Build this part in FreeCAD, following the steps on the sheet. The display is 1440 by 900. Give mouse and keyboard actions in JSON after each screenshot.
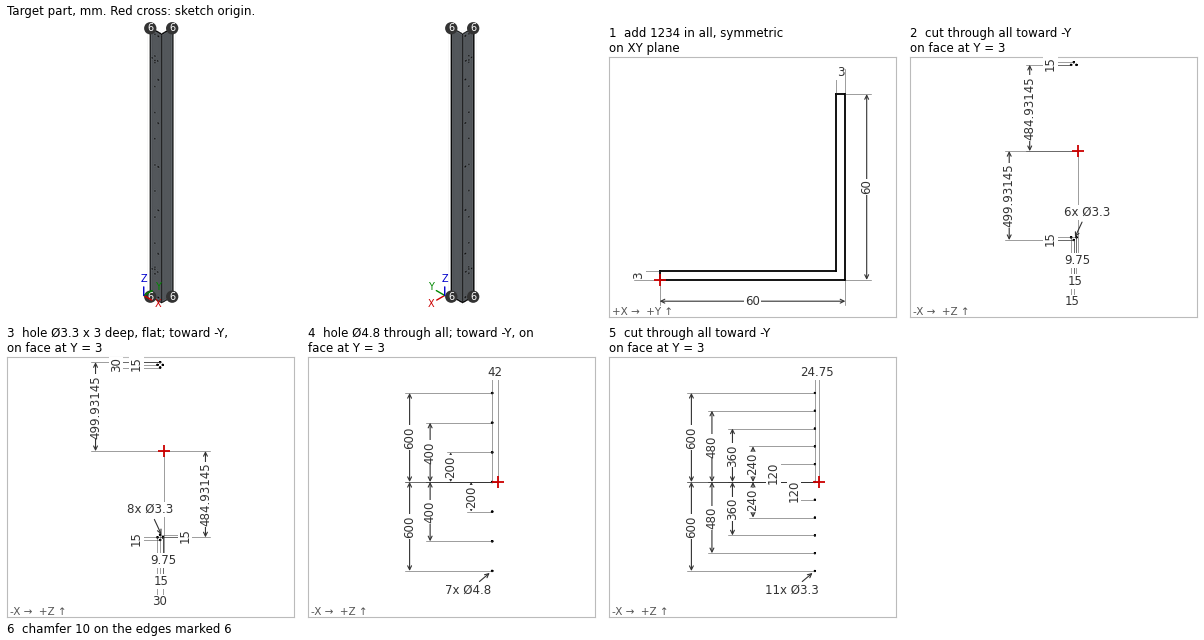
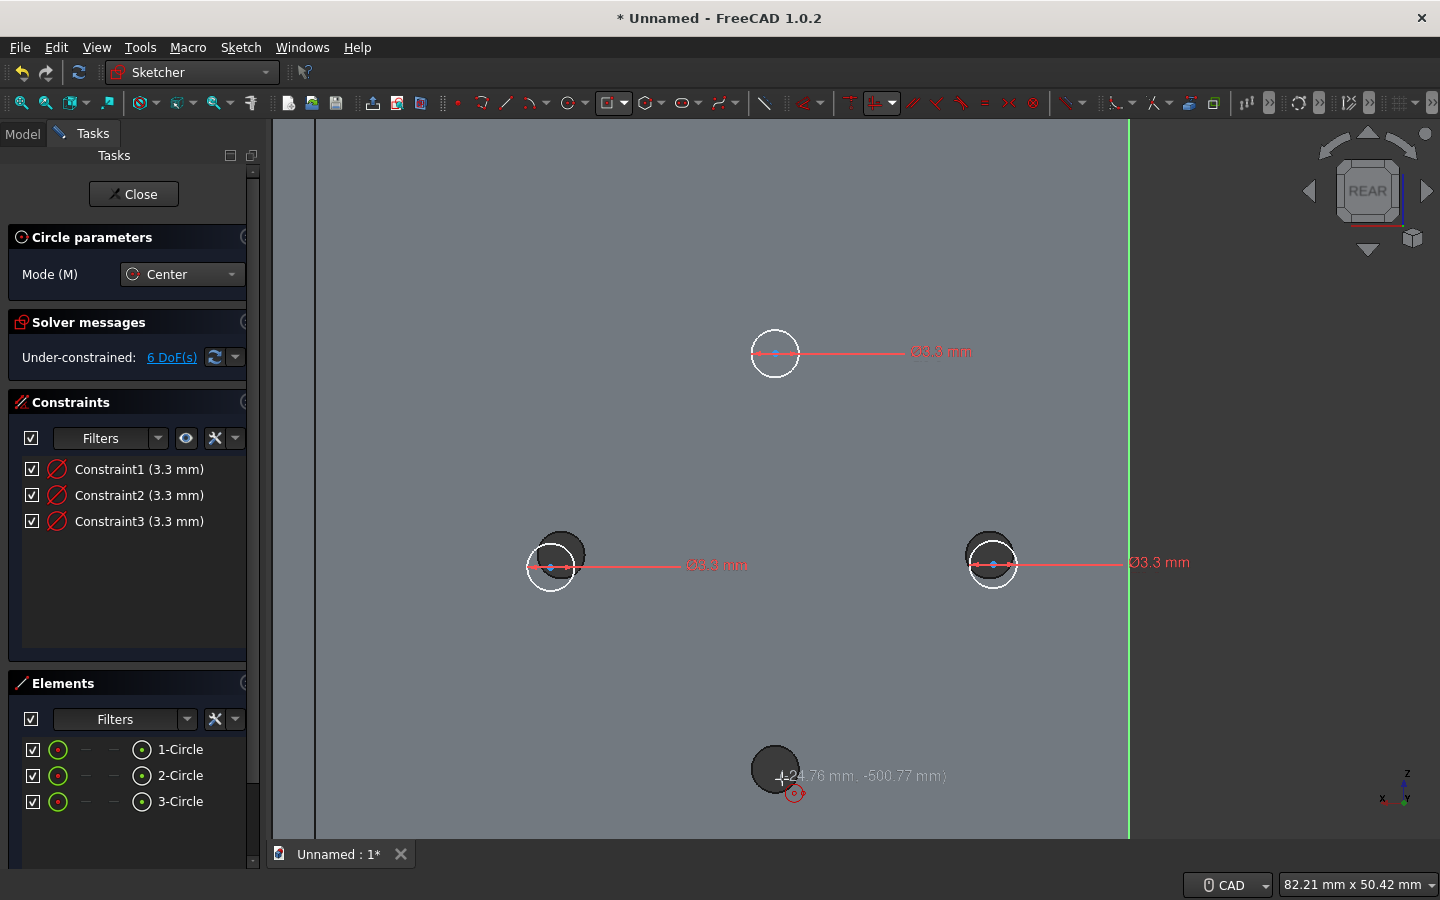
{"action": "scroll", "coordinate": [782, 770], "scroll_direction": "down", "scroll_amount": 16}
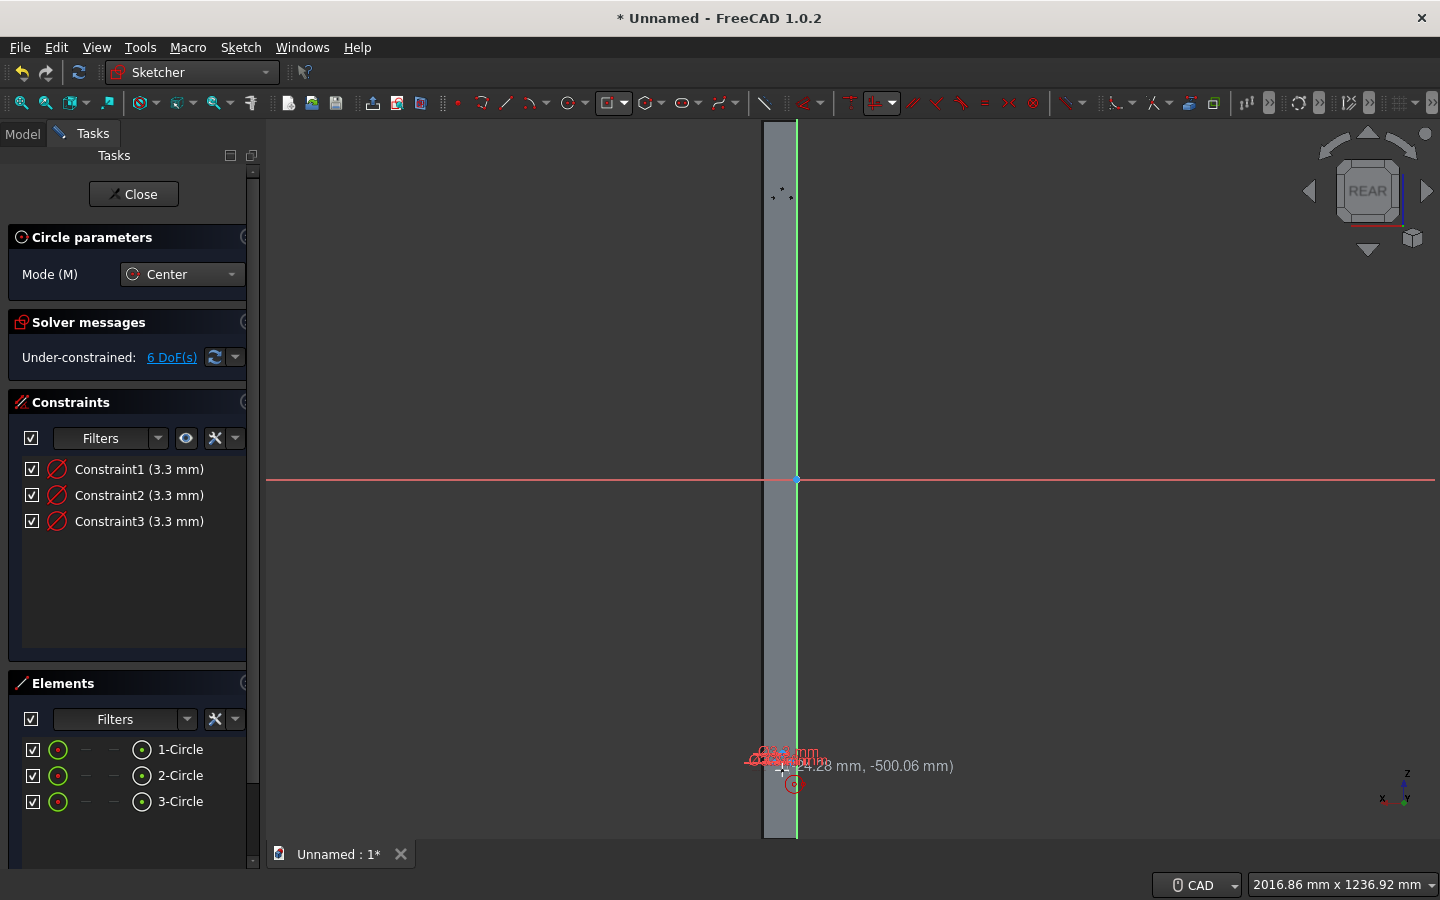
{"action": "scroll", "coordinate": [782, 771], "scroll_direction": "up", "scroll_amount": 2}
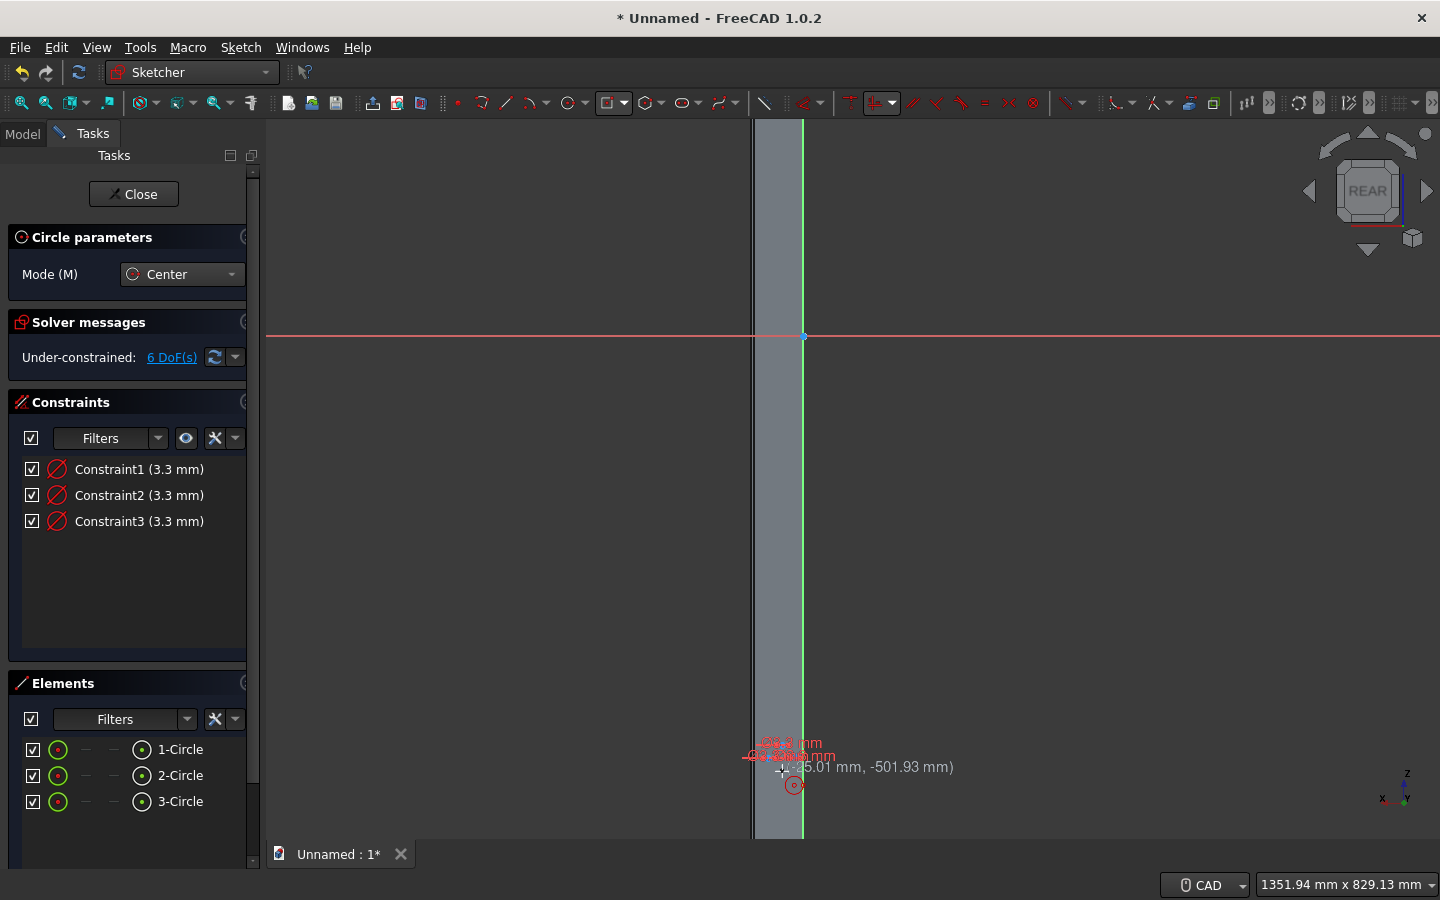
{"action": "left_click", "coordinate": [782, 770]}
{"action": "mouse_move", "coordinate": [783, 769]}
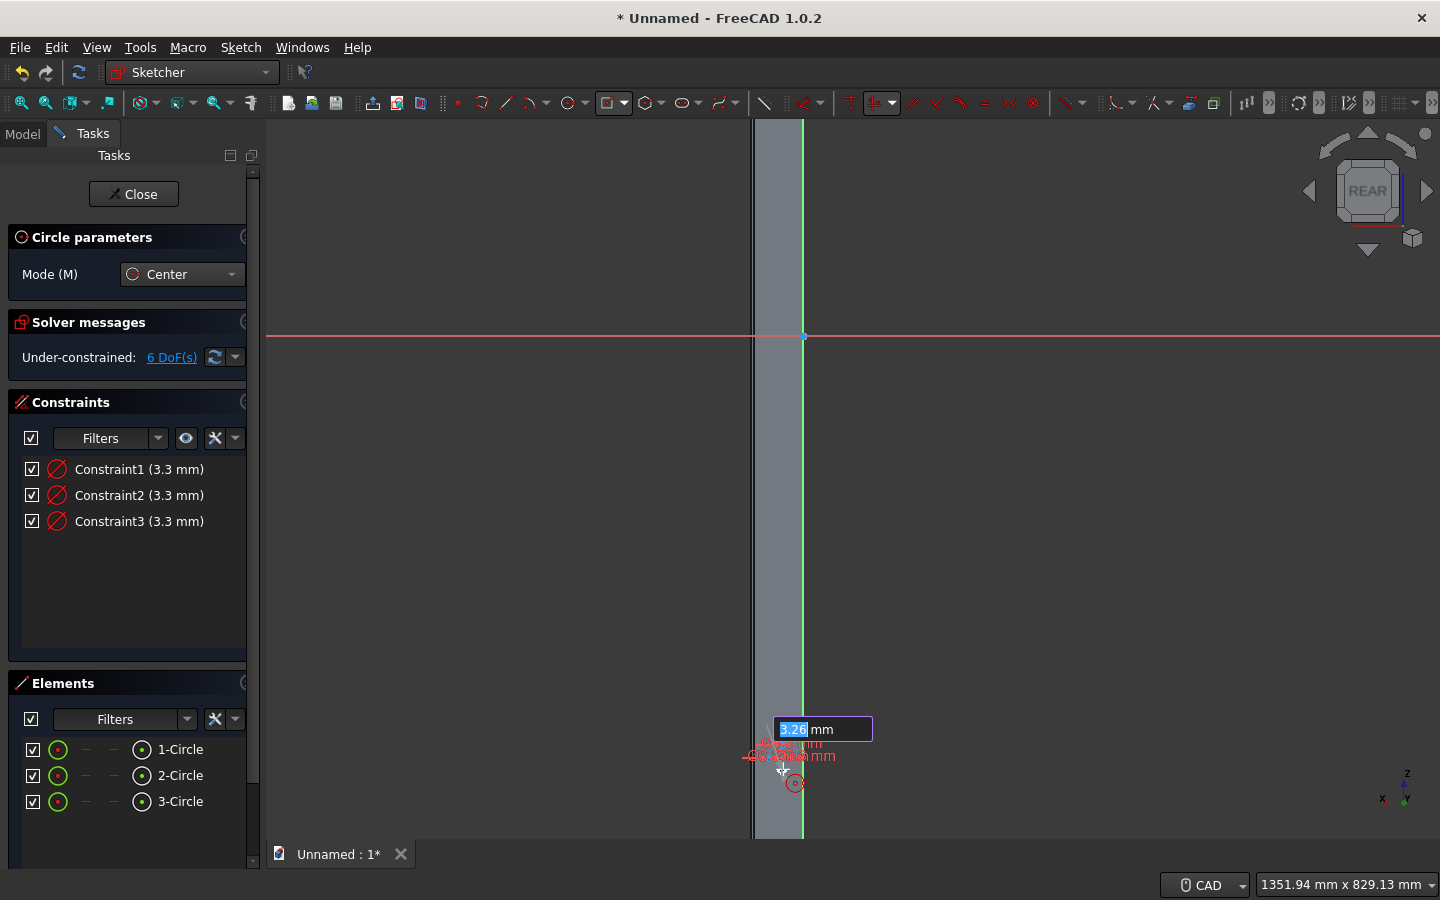
{"action": "type", "text": "3.3"}
{"action": "key", "text": "Return"}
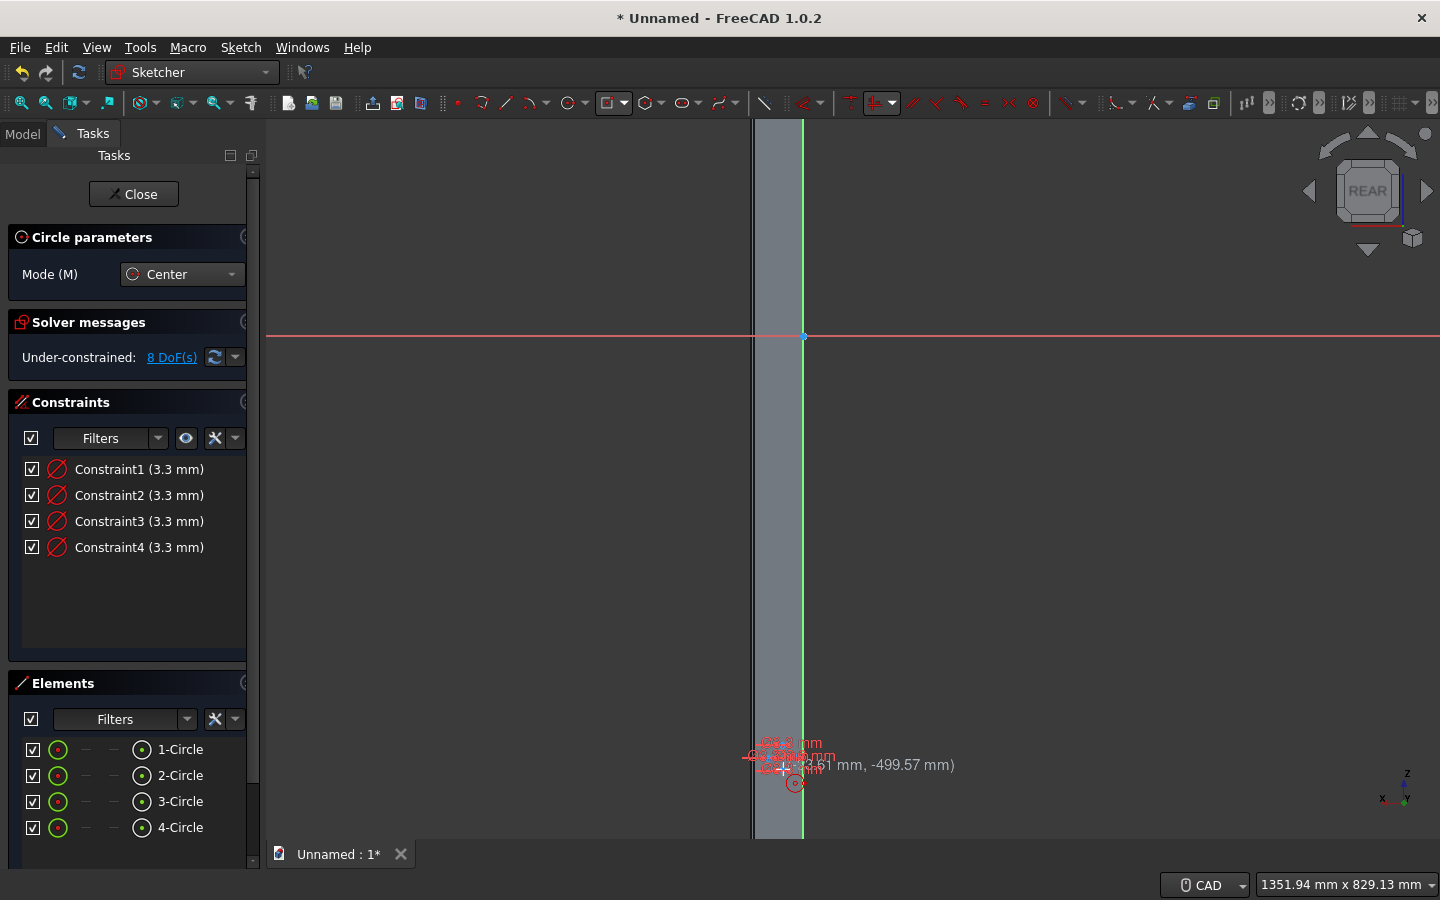
{"action": "scroll", "coordinate": [783, 653], "scroll_direction": "down", "scroll_amount": 3}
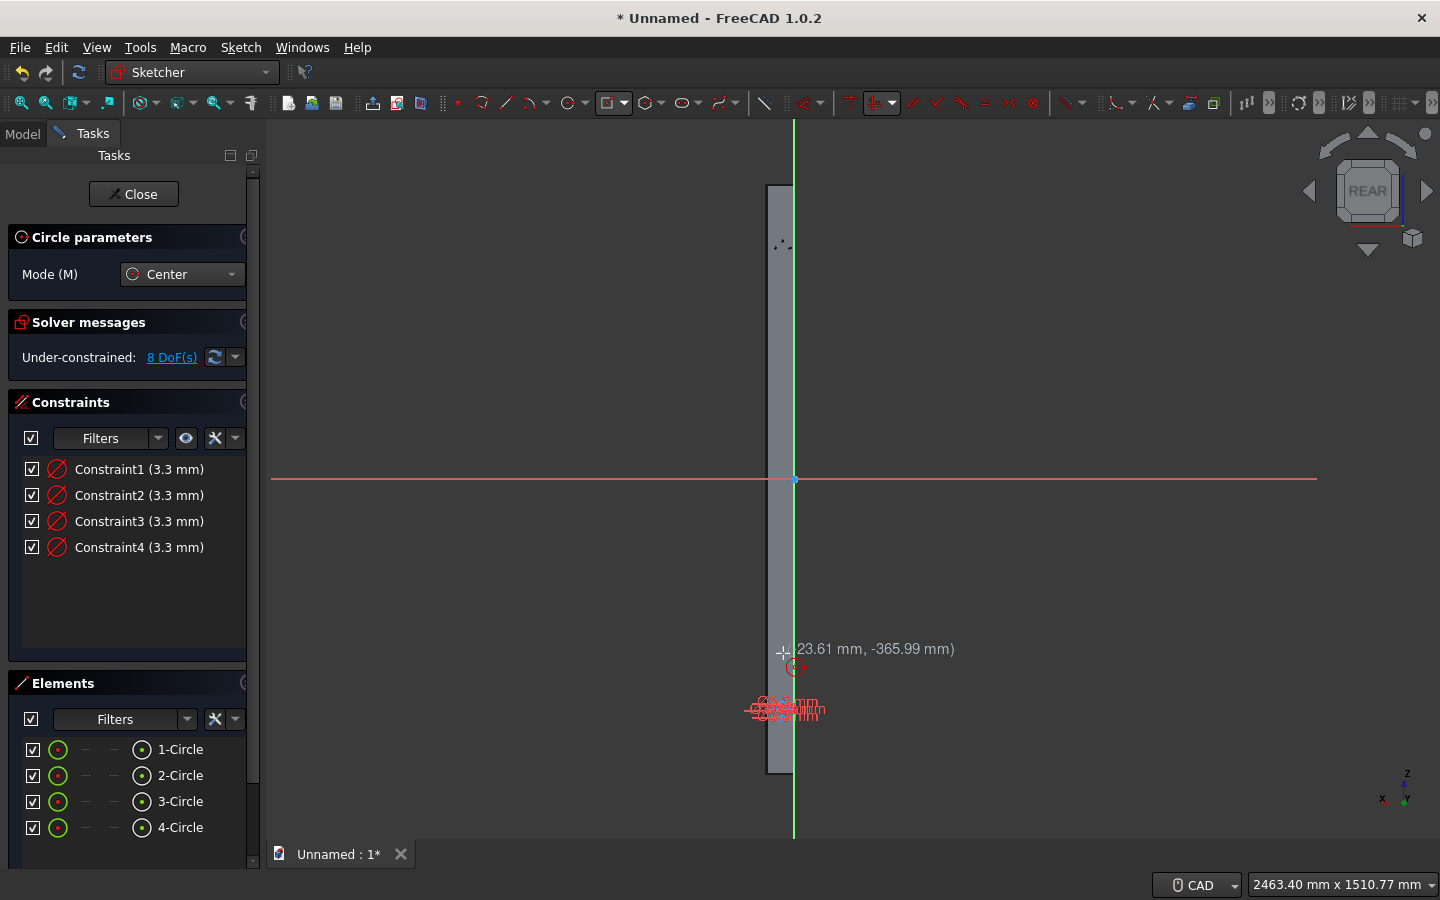
{"action": "scroll", "coordinate": [783, 241], "scroll_direction": "up", "scroll_amount": 17}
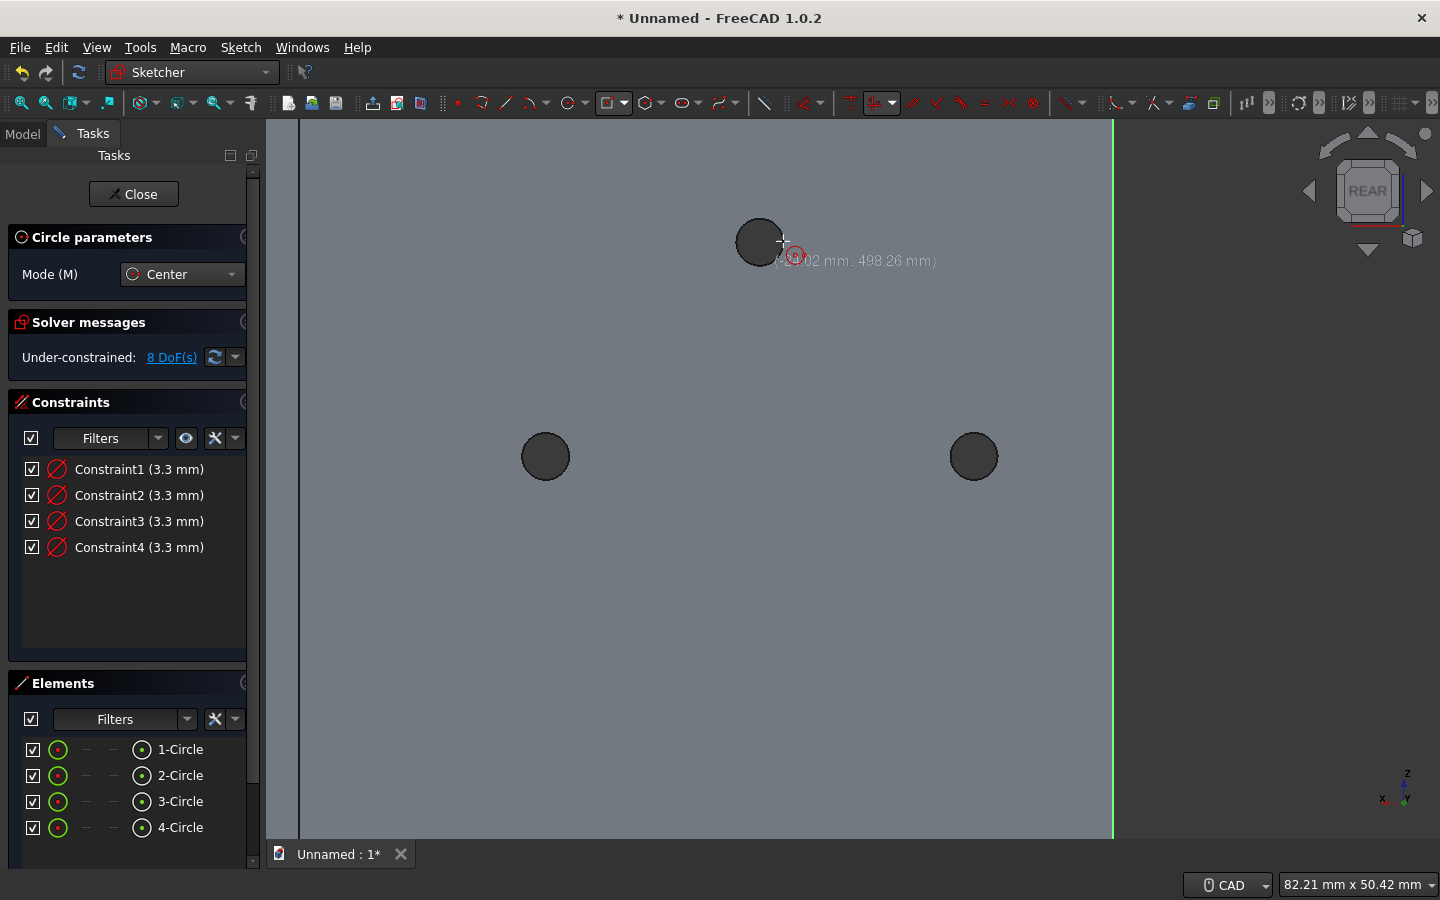
{"action": "scroll", "coordinate": [783, 186], "scroll_direction": "down", "scroll_amount": 16}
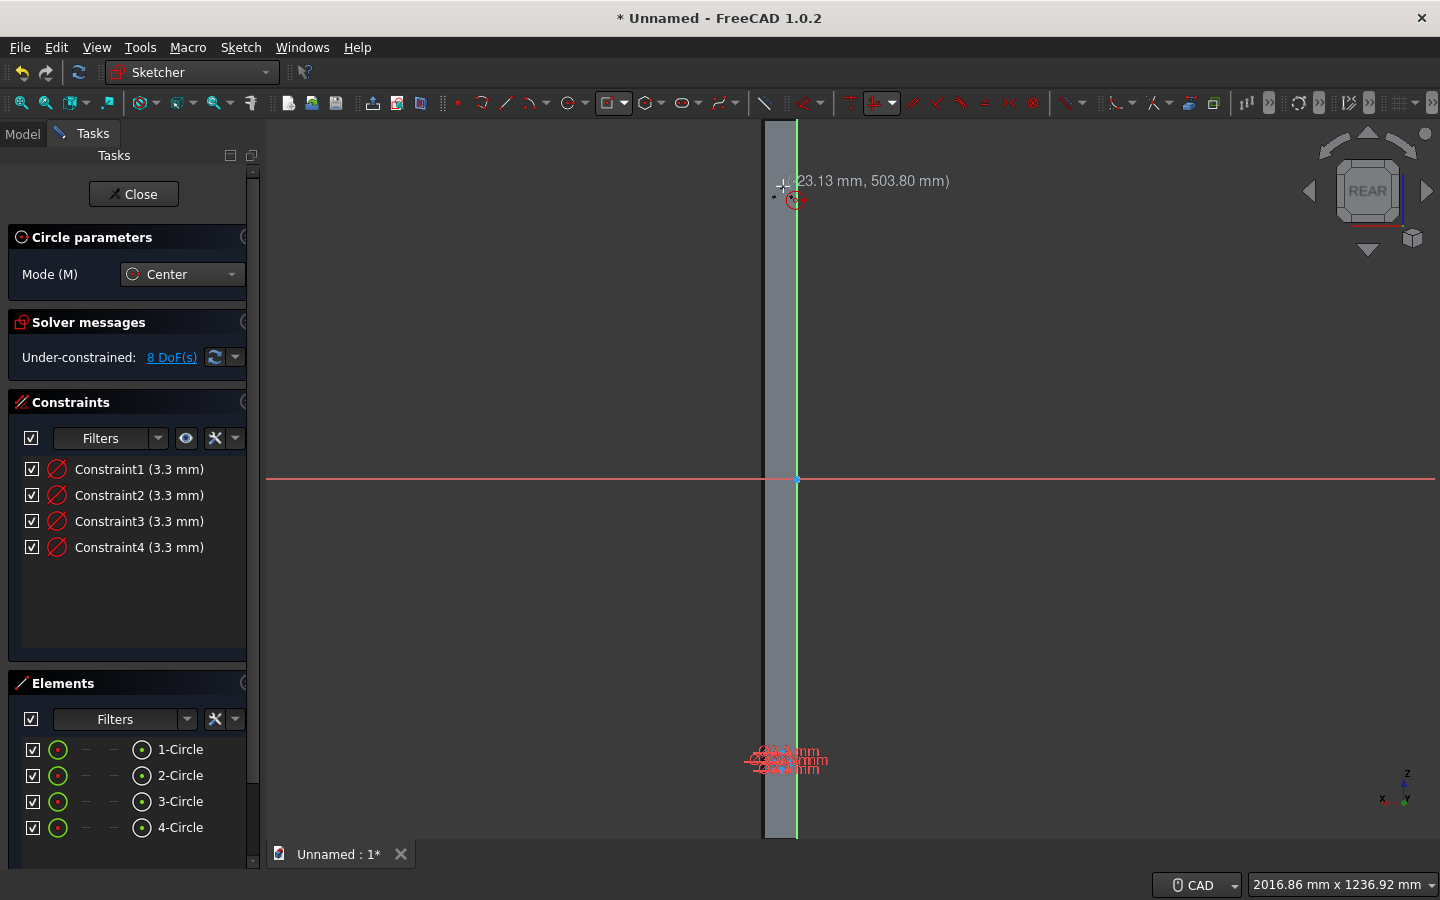
{"action": "left_click", "coordinate": [782, 188]}
{"action": "mouse_move", "coordinate": [782, 188]}